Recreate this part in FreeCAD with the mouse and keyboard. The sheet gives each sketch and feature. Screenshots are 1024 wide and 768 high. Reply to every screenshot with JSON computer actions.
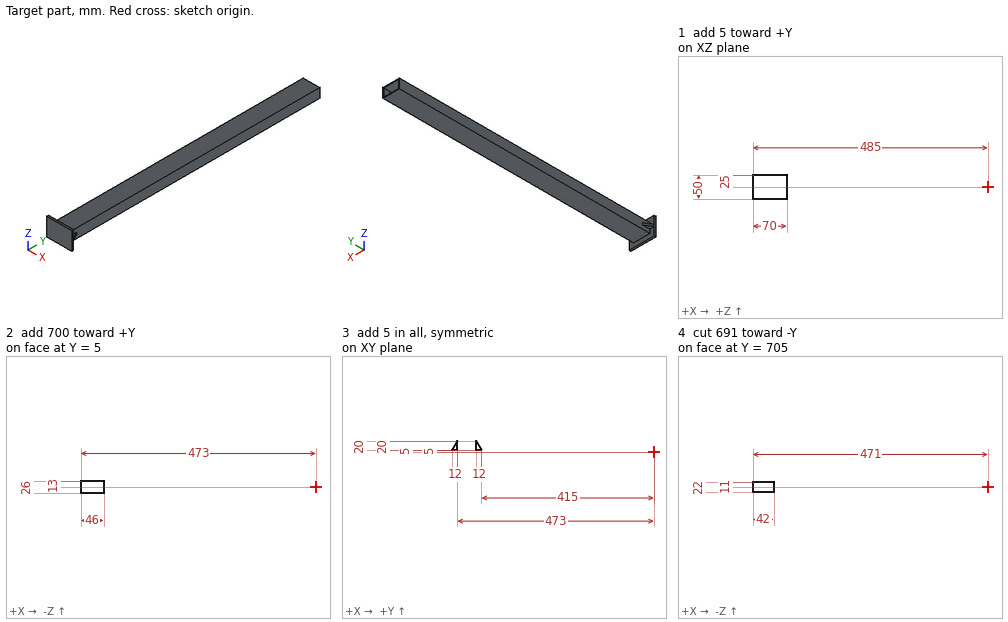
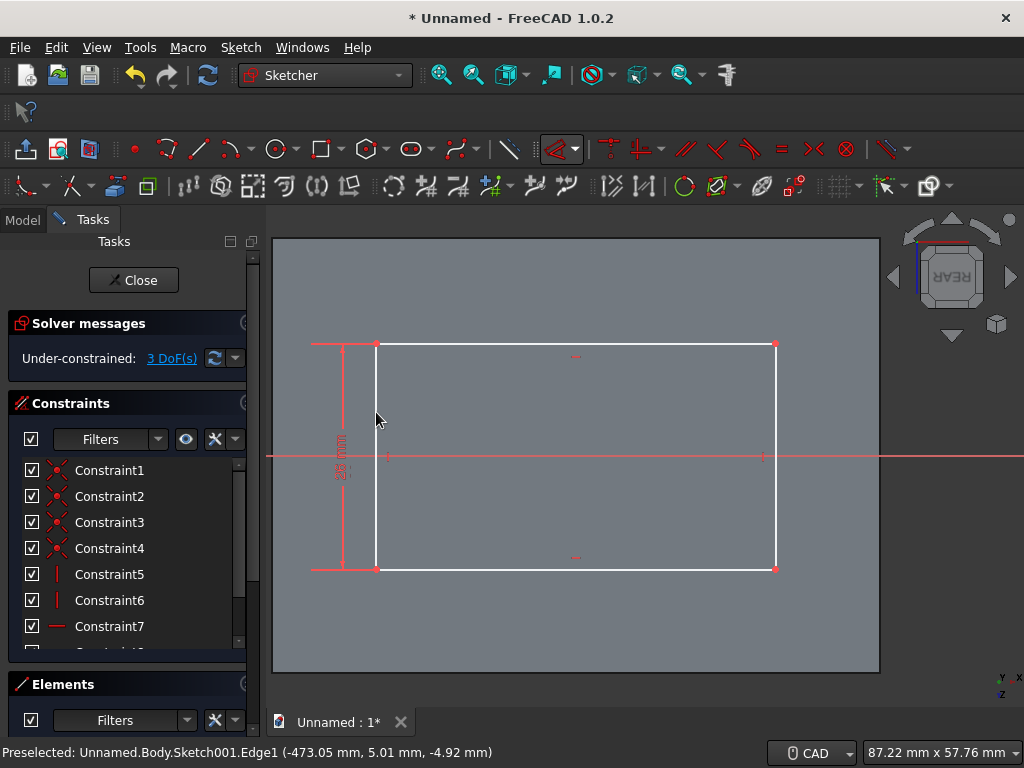
{"action": "left_click", "coordinate": [496, 570]}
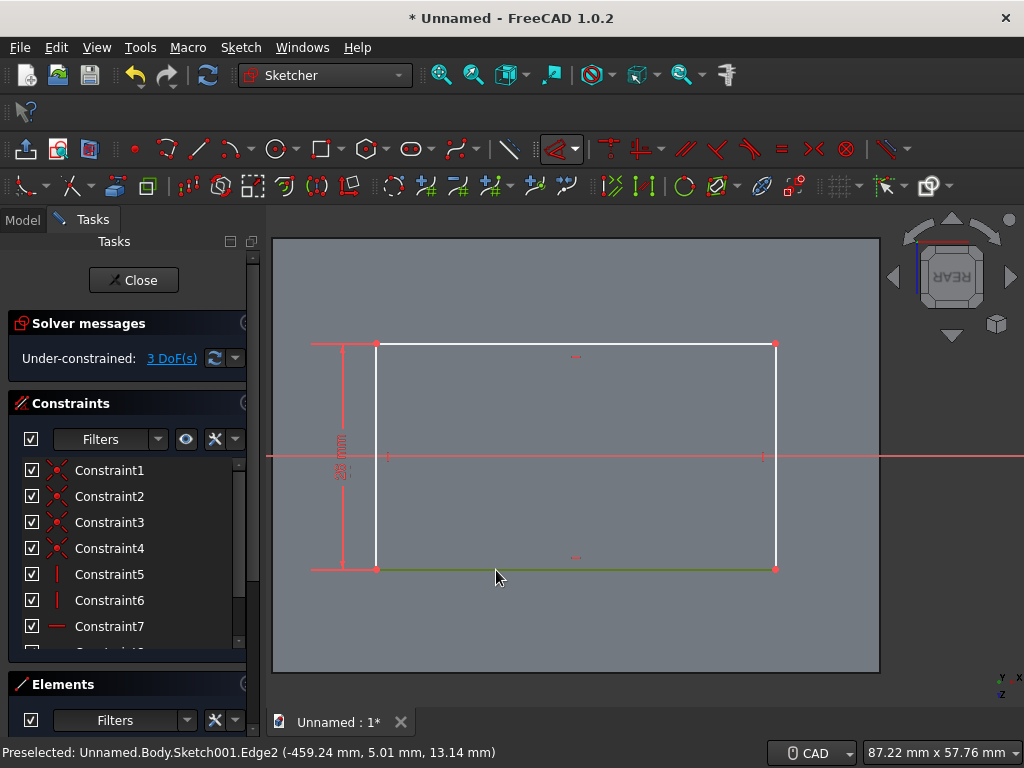
{"action": "left_click", "coordinate": [578, 150]}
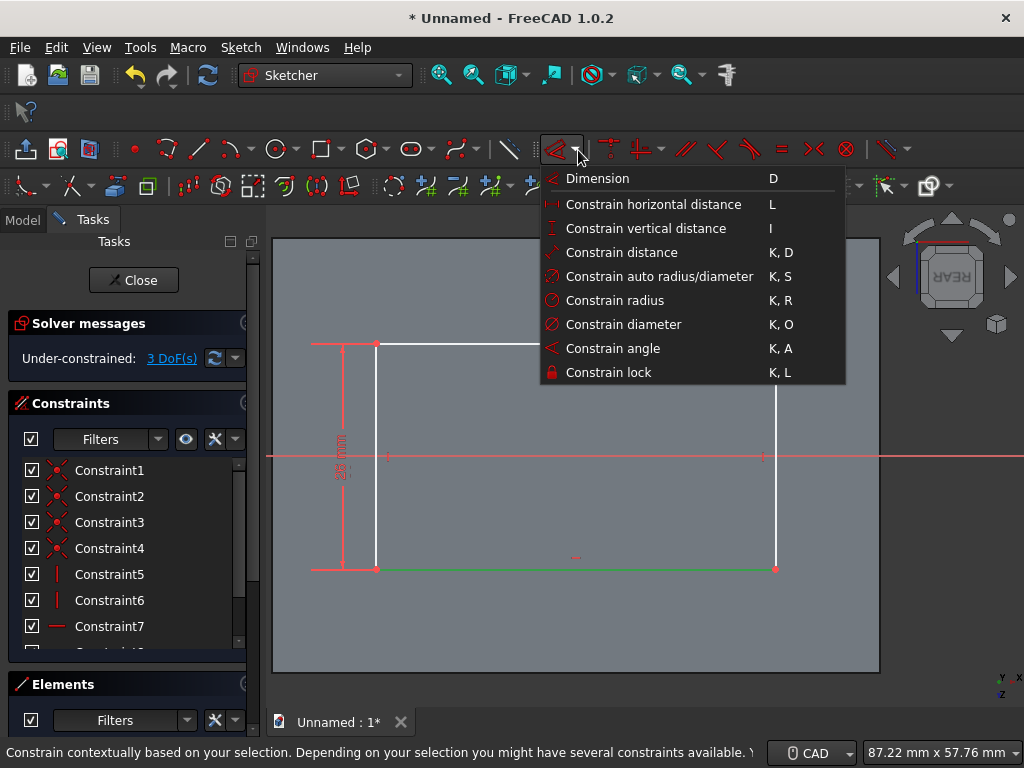
{"action": "left_click", "coordinate": [693, 204]}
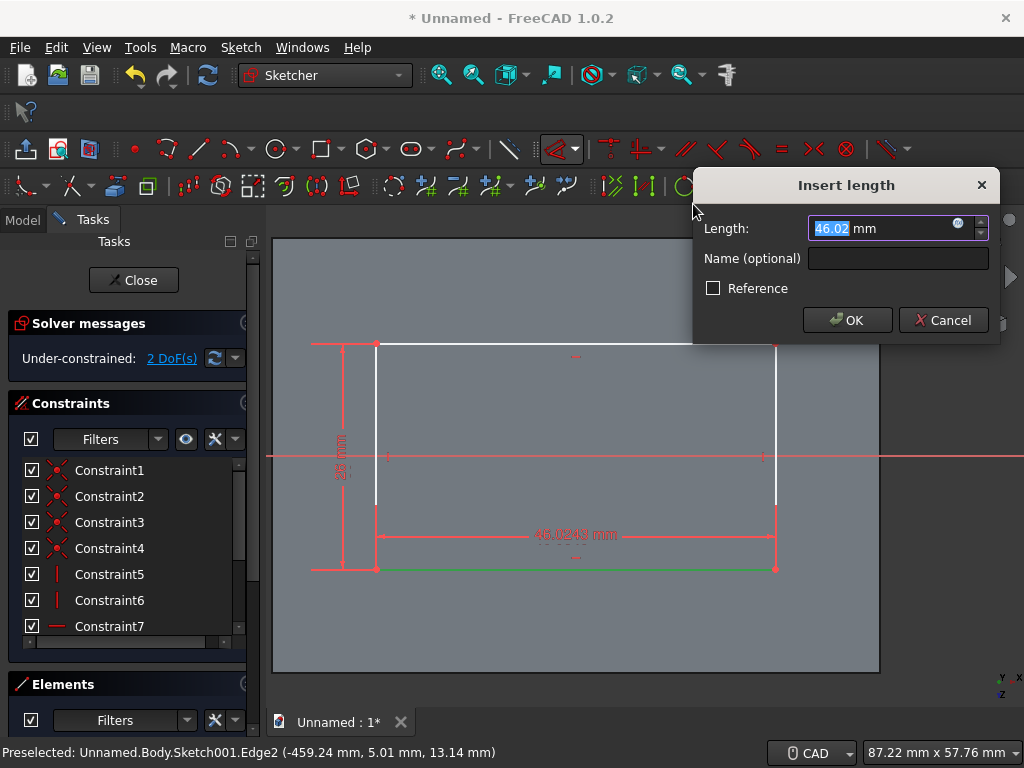
{"action": "type", "text": "46"}
{"action": "key", "text": "Return"}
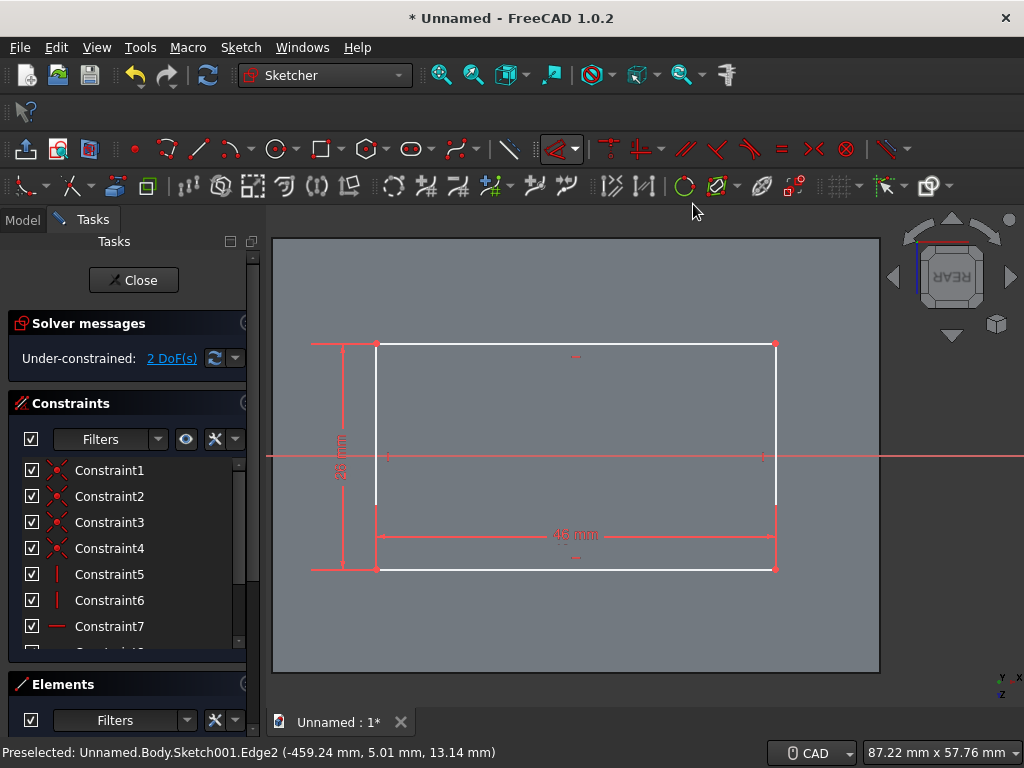
{"action": "left_click", "coordinate": [376, 344]}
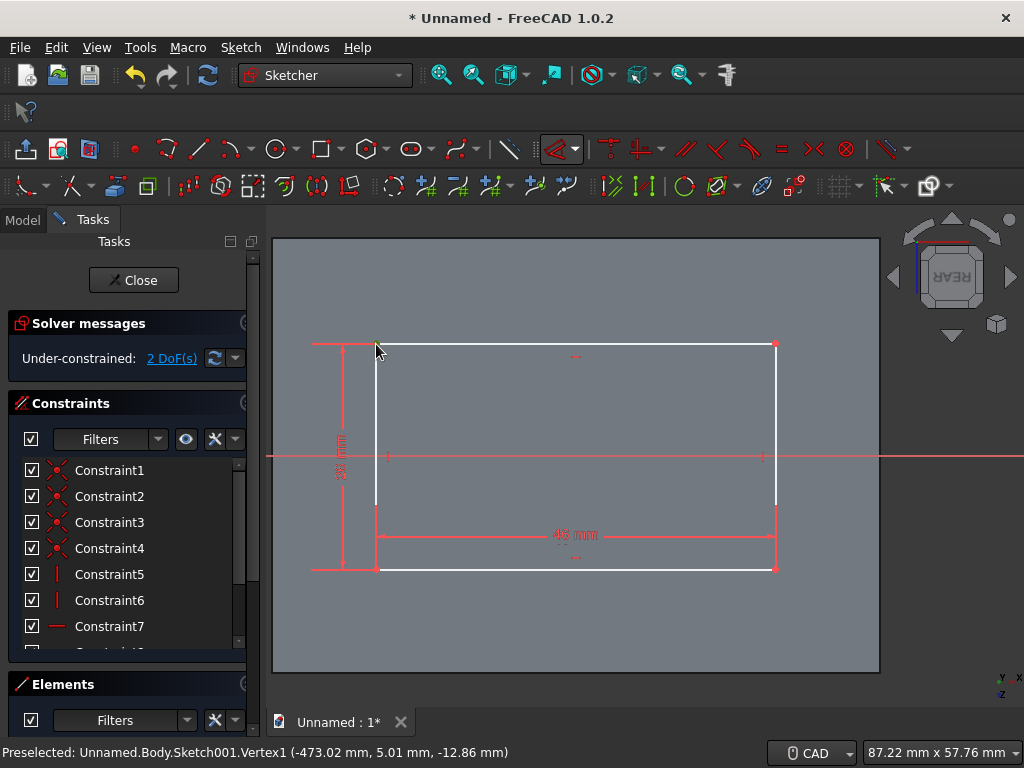
{"action": "left_click", "coordinate": [578, 150]}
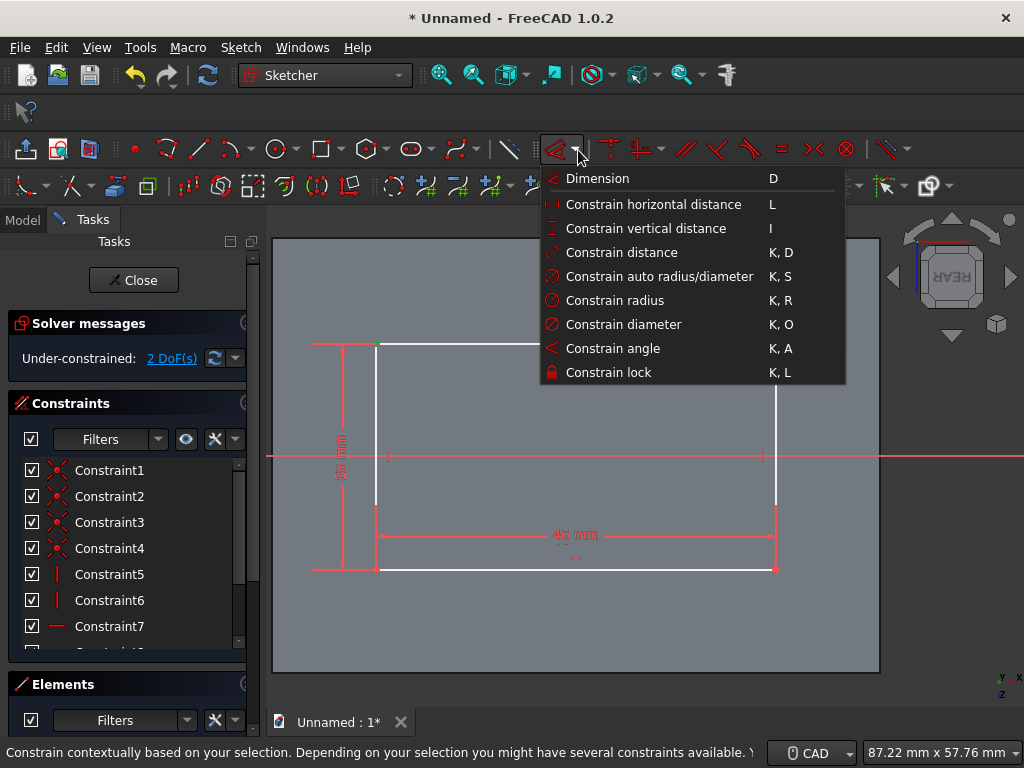
{"action": "left_click", "coordinate": [693, 228]}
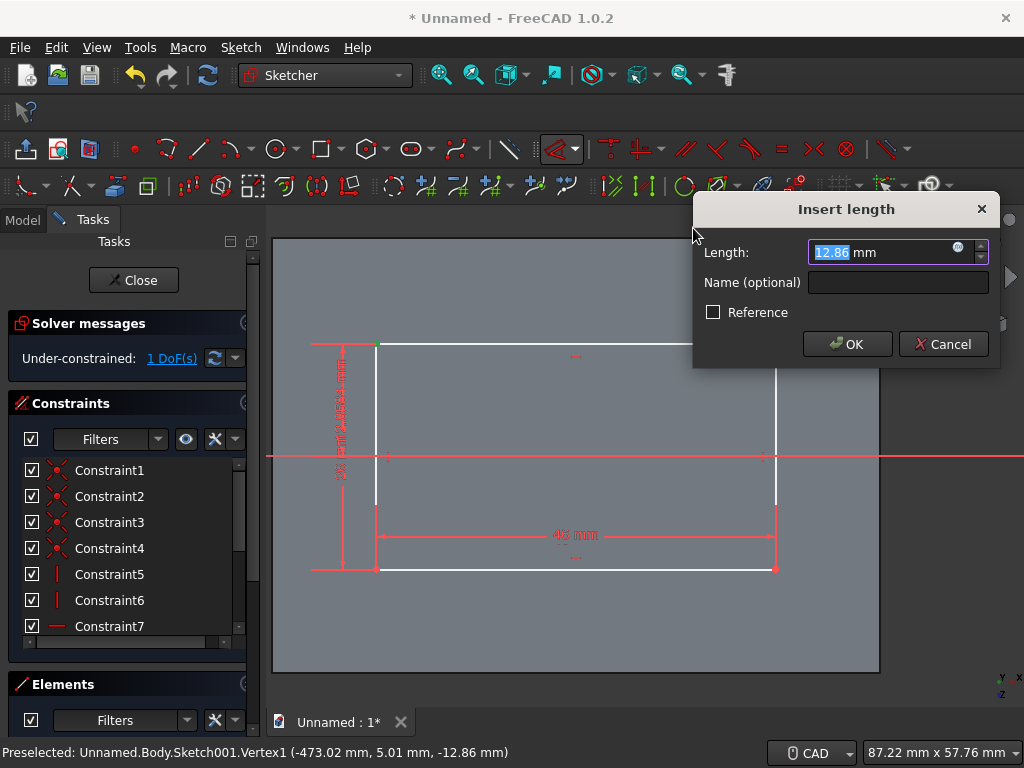
{"action": "type", "text": "13"}
{"action": "key", "text": "Return"}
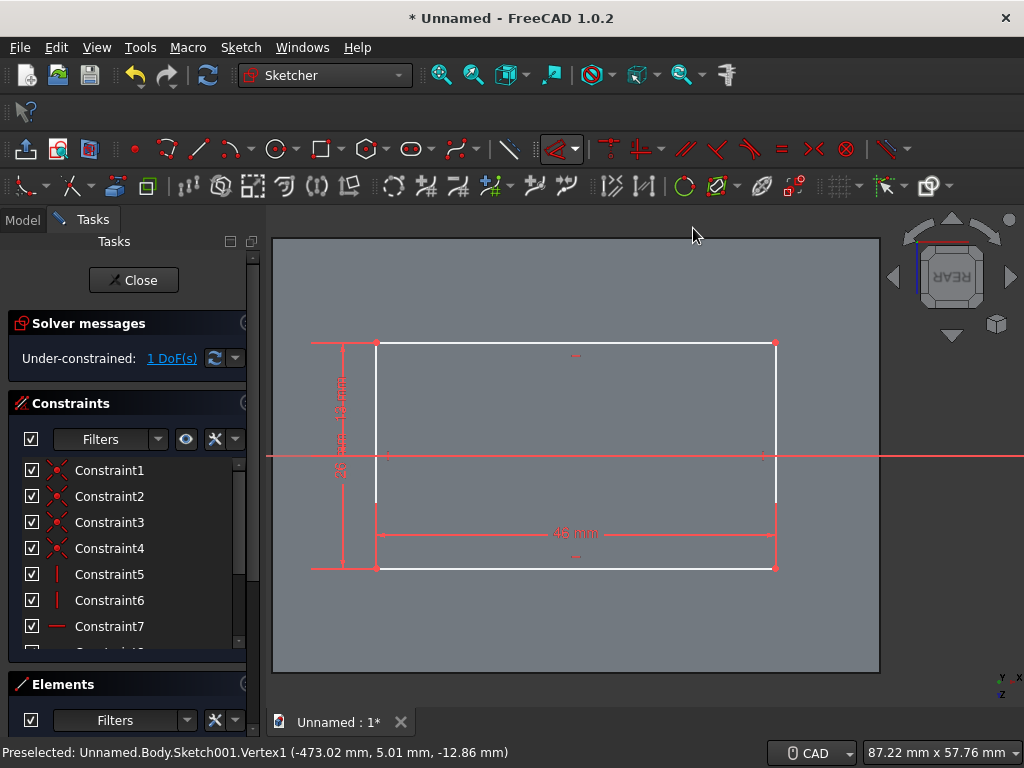
{"action": "left_click", "coordinate": [376, 343]}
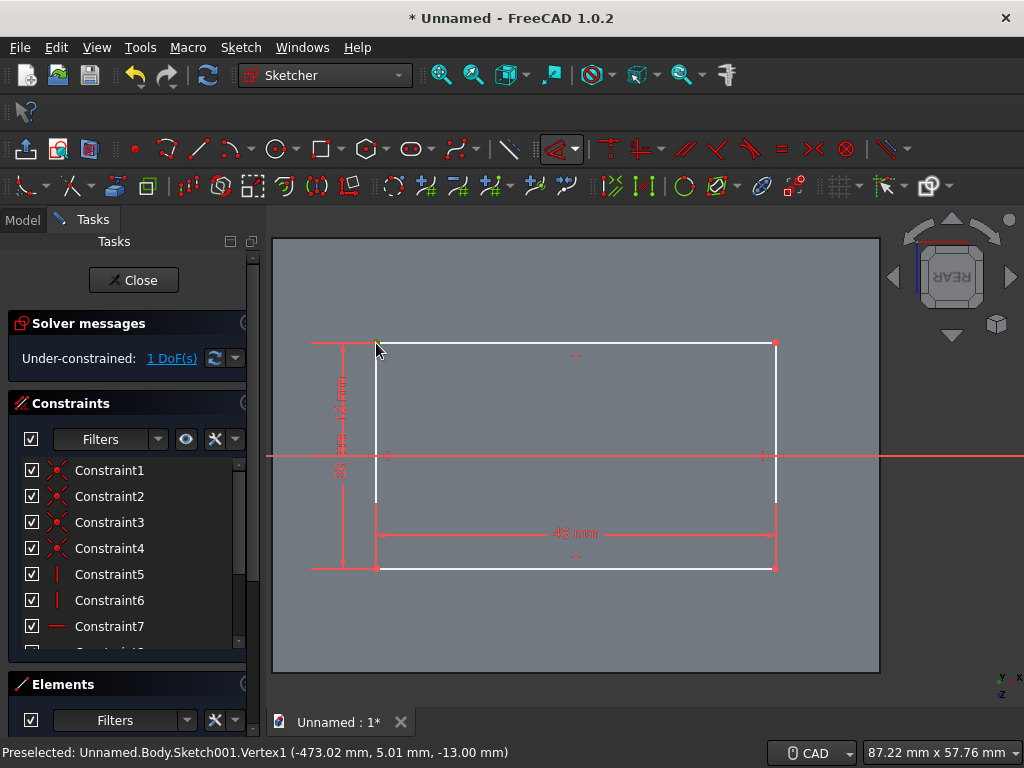
{"action": "left_click", "coordinate": [578, 150]}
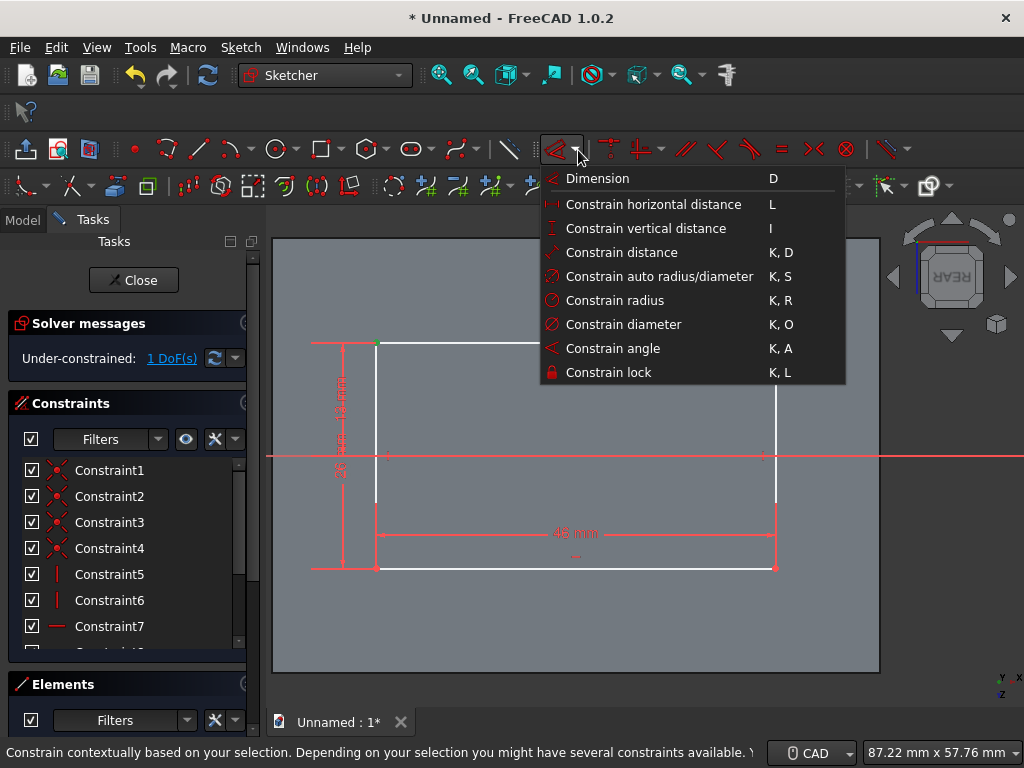
{"action": "left_click", "coordinate": [693, 204]}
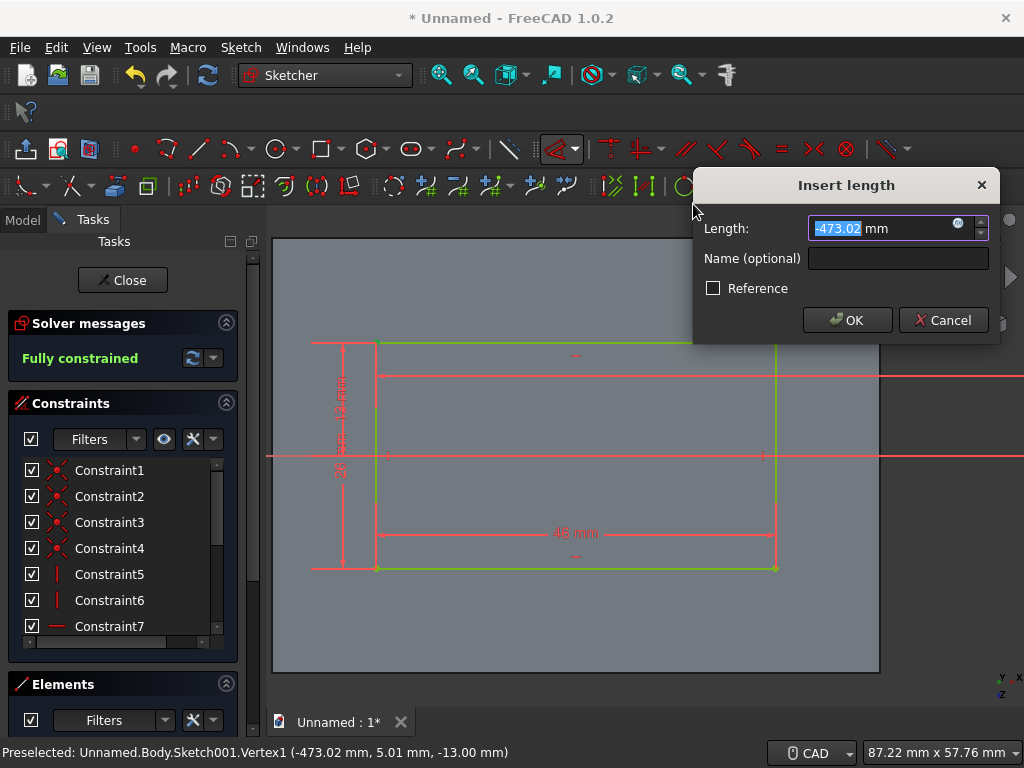
{"action": "type", "text": "-473"}
{"action": "key", "text": "Return"}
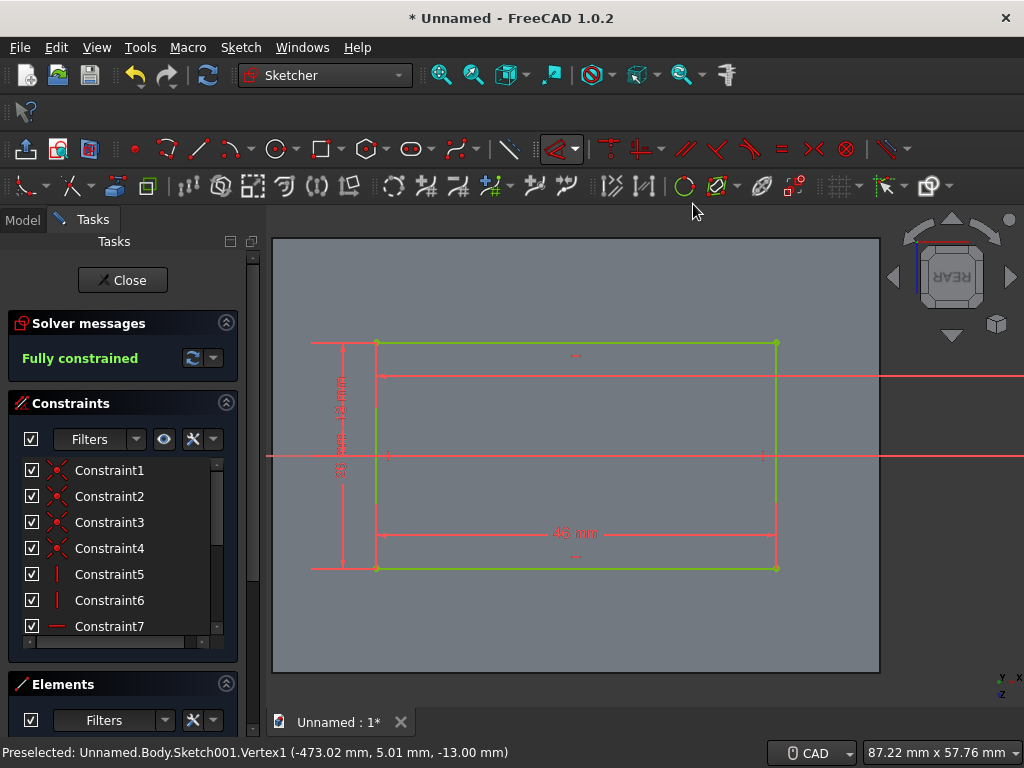
{"action": "left_click", "coordinate": [123, 280]}